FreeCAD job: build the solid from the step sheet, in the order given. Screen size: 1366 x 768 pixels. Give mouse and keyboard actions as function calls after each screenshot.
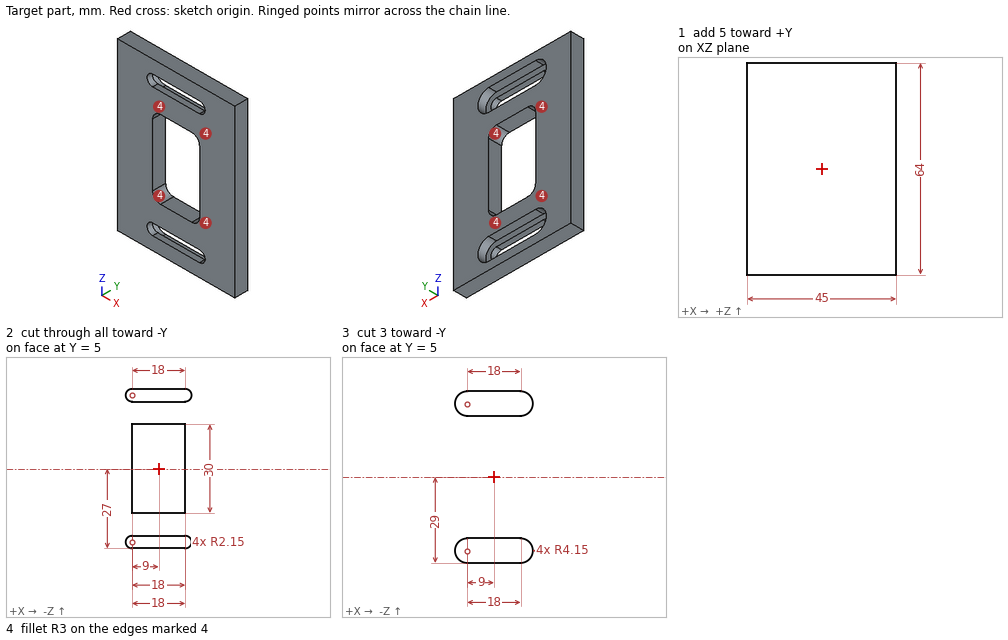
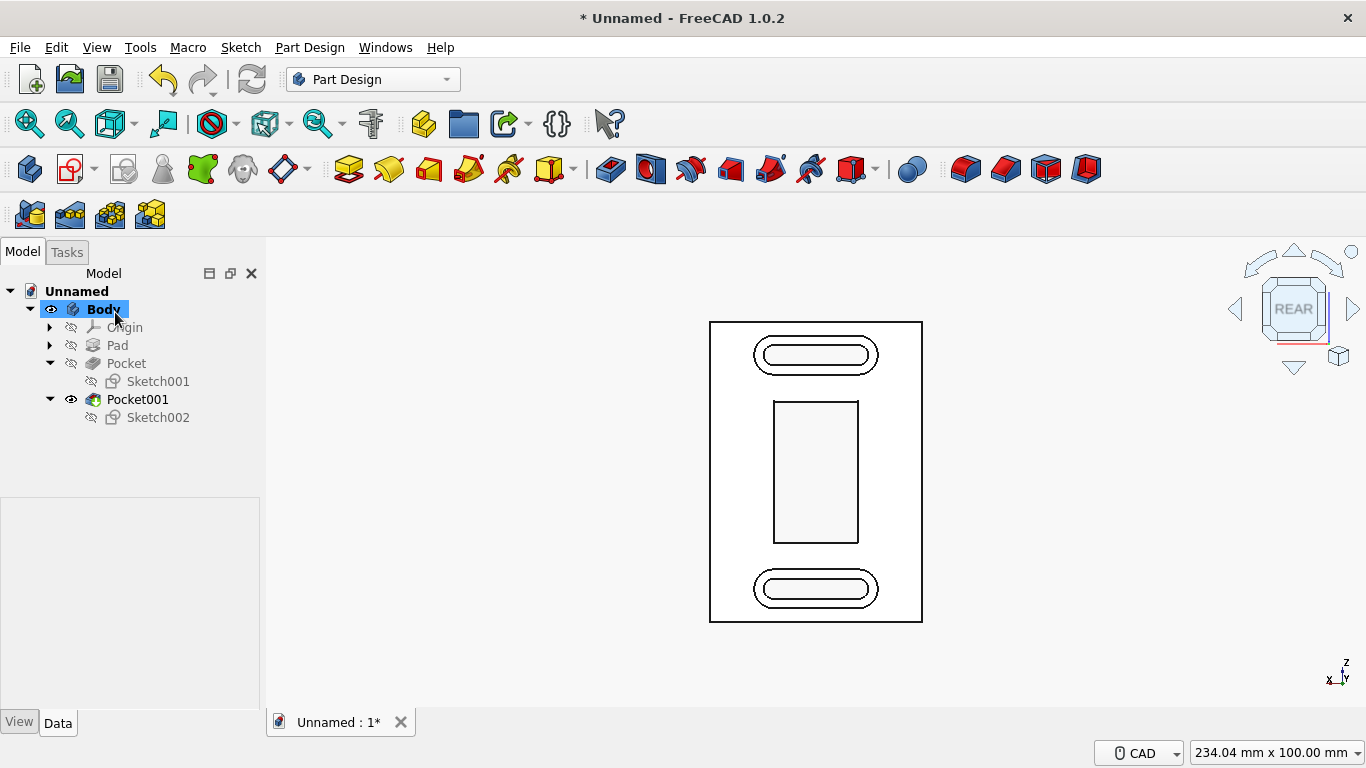
key(0)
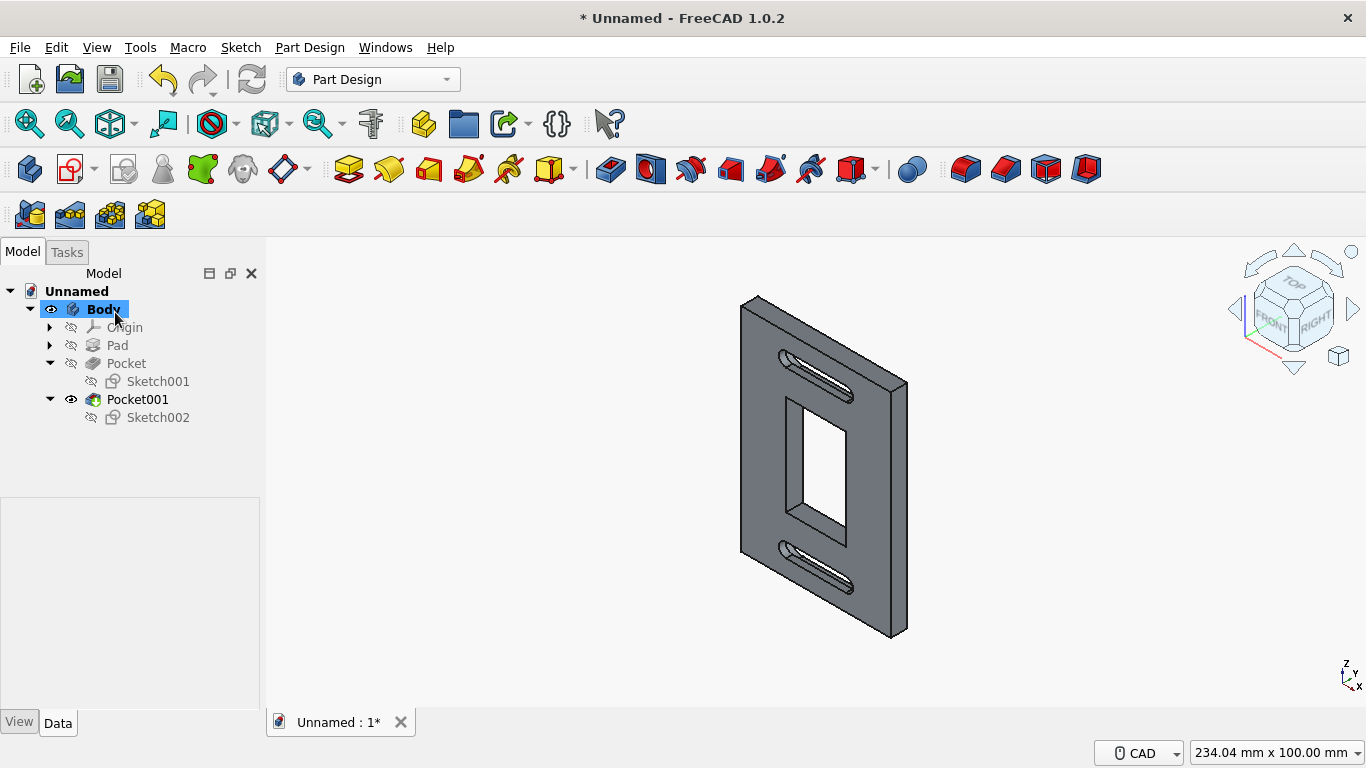
key(2)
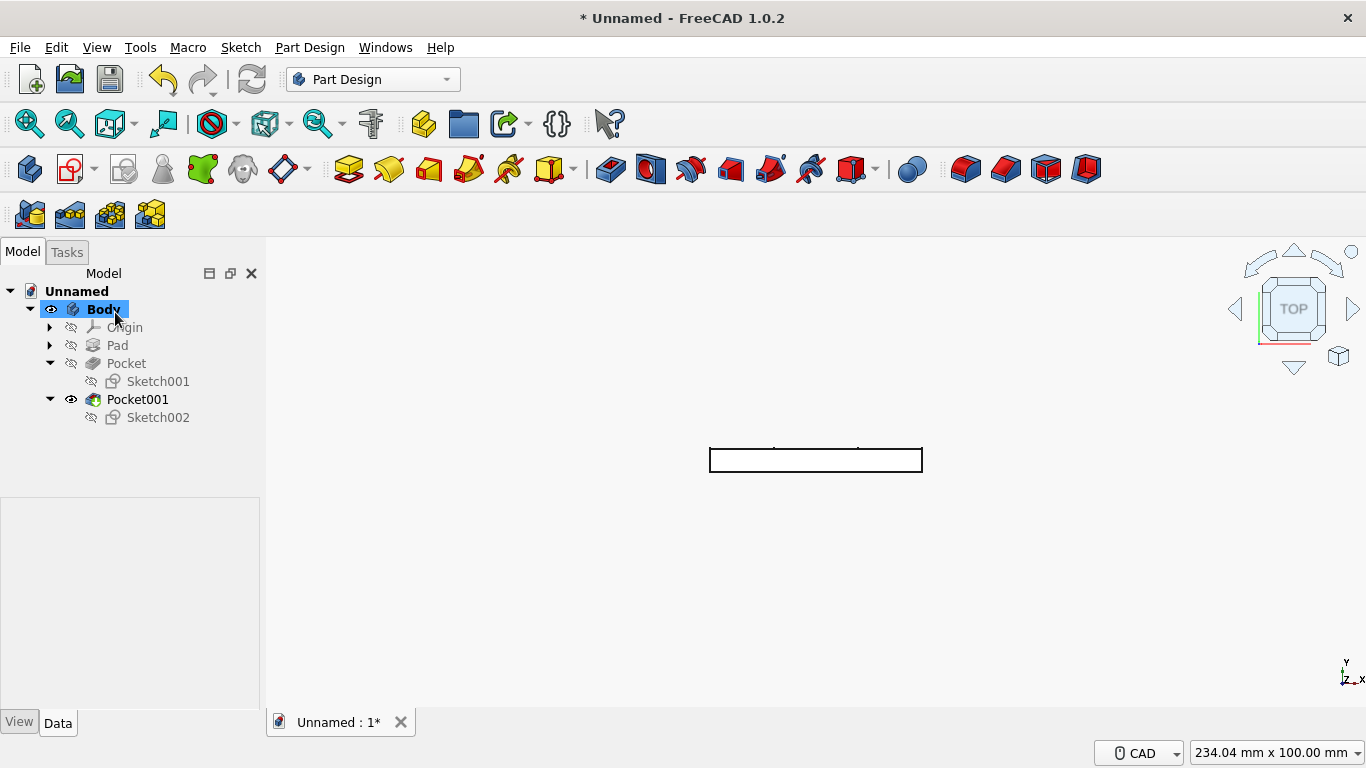
click(30, 124)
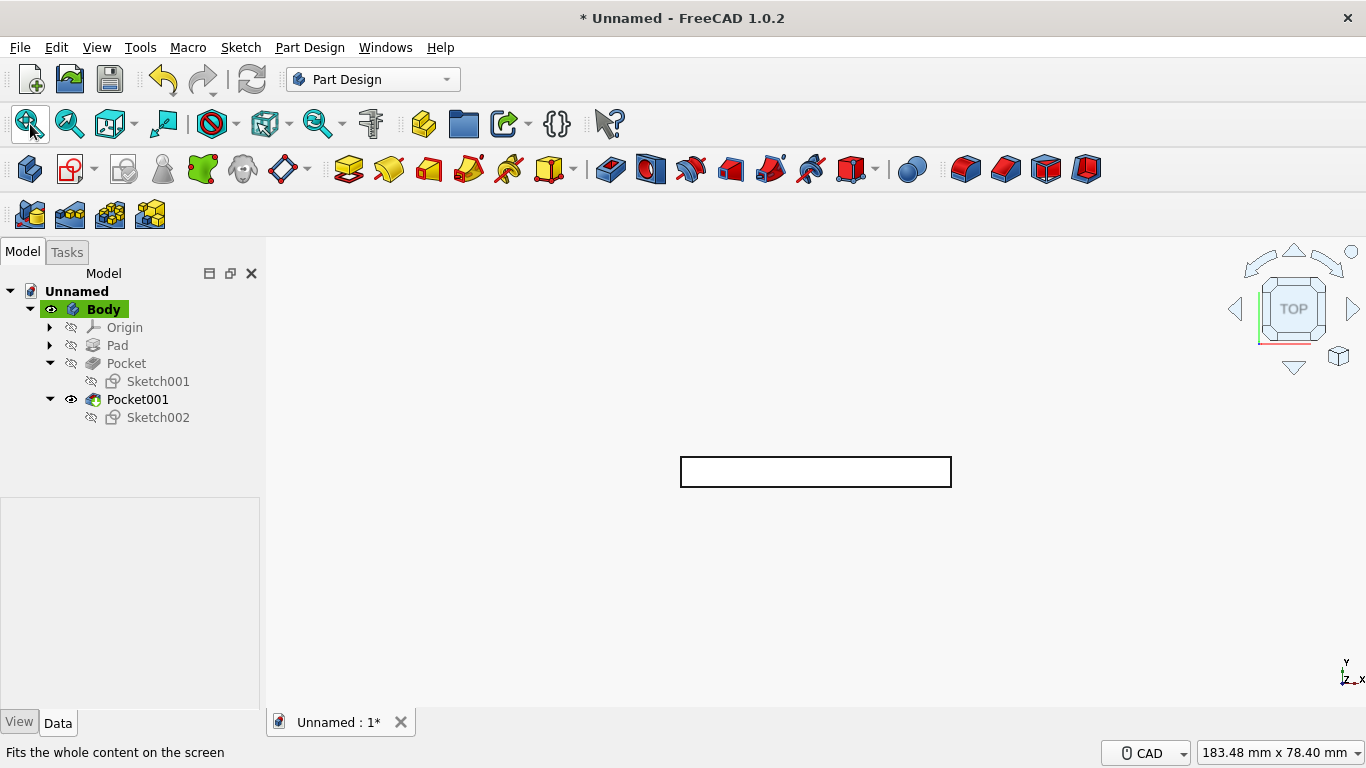
key(1)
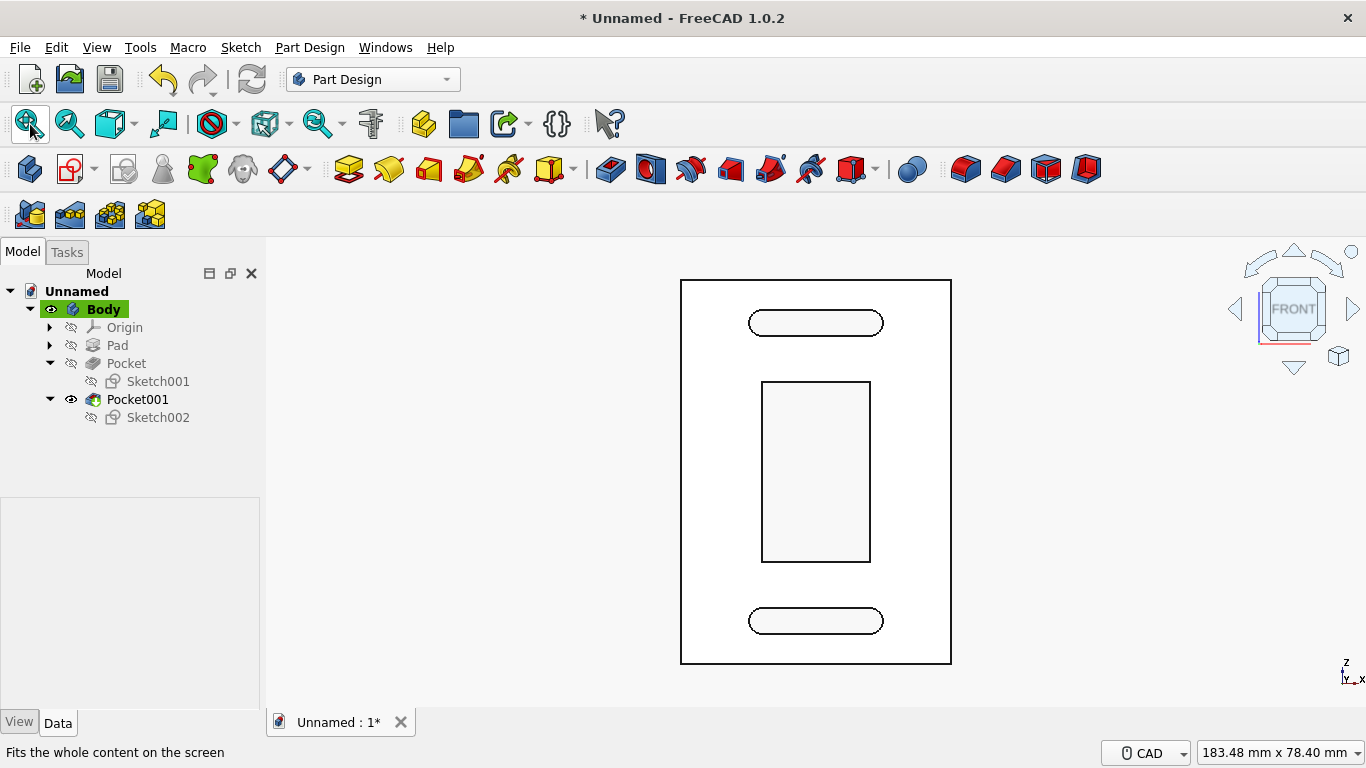
key(3)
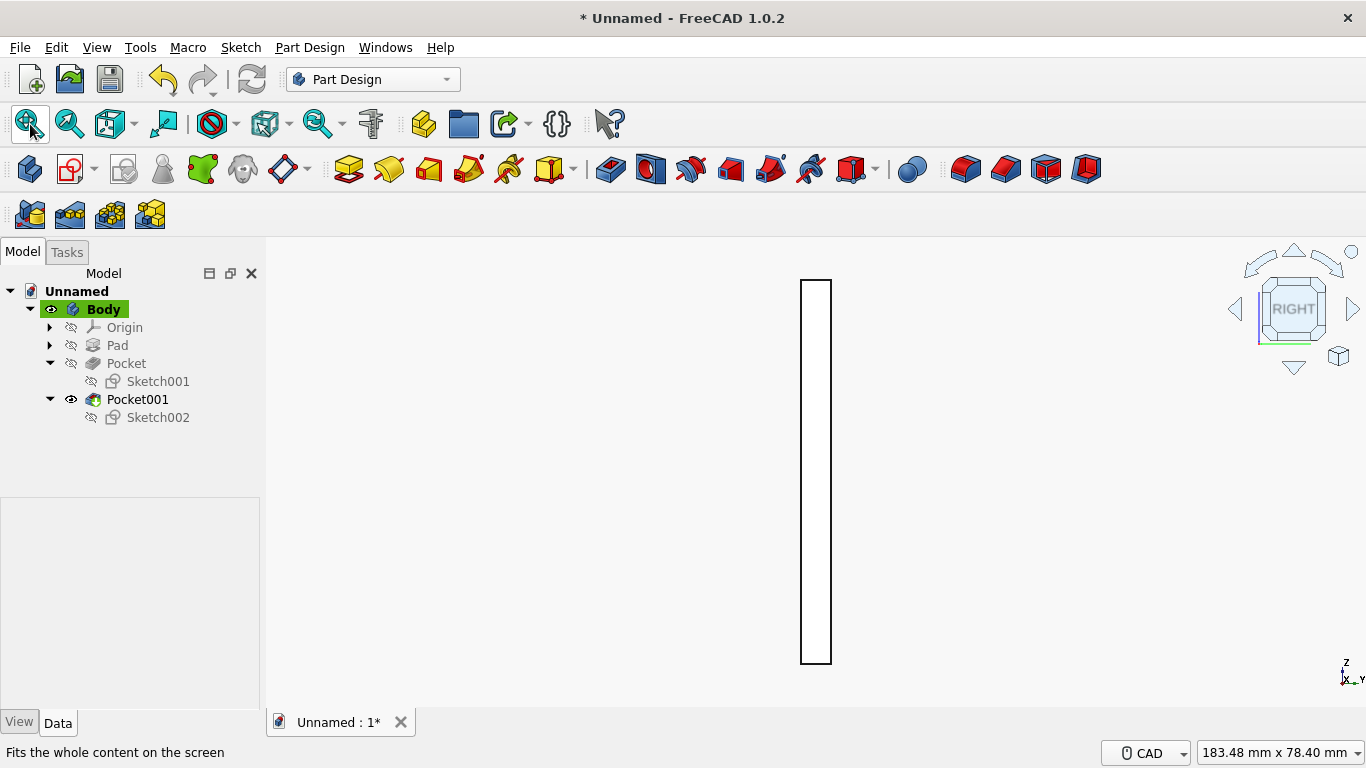
key(5)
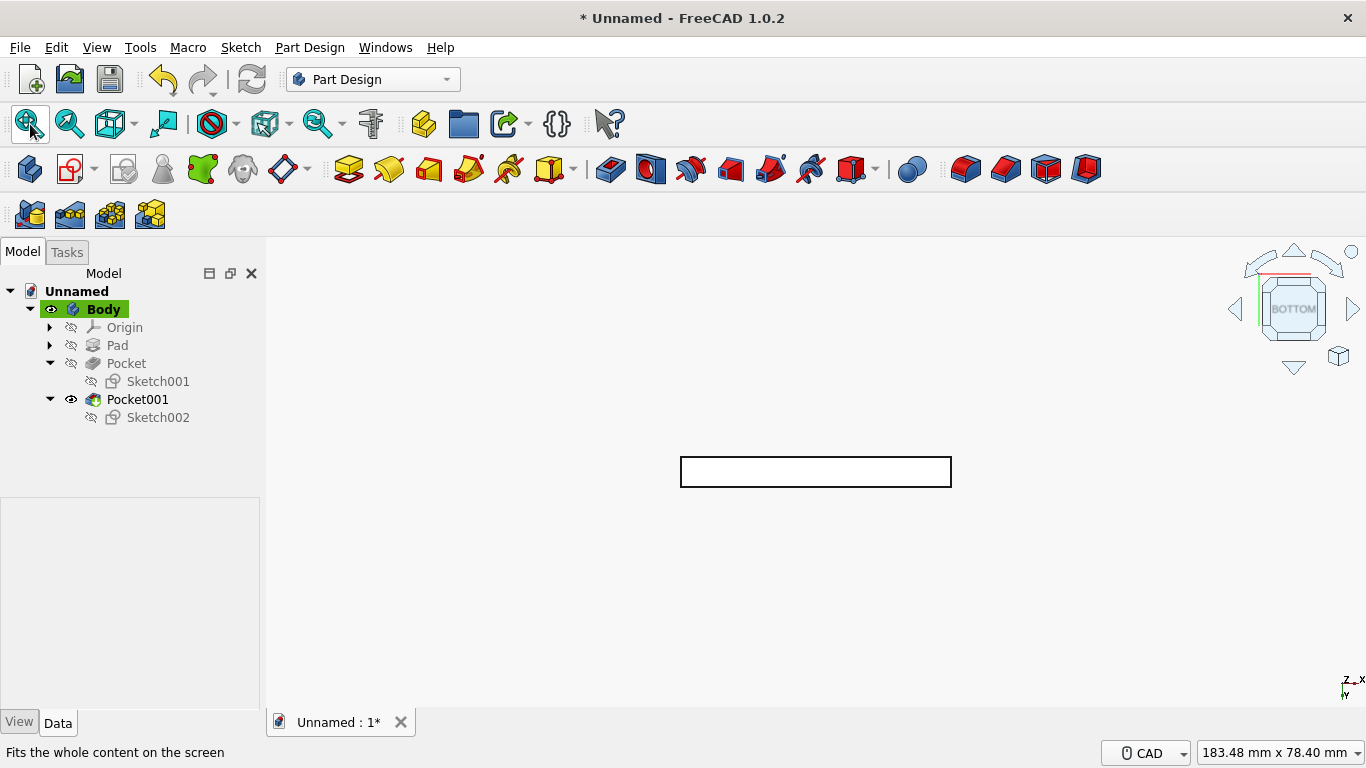
click(30, 124)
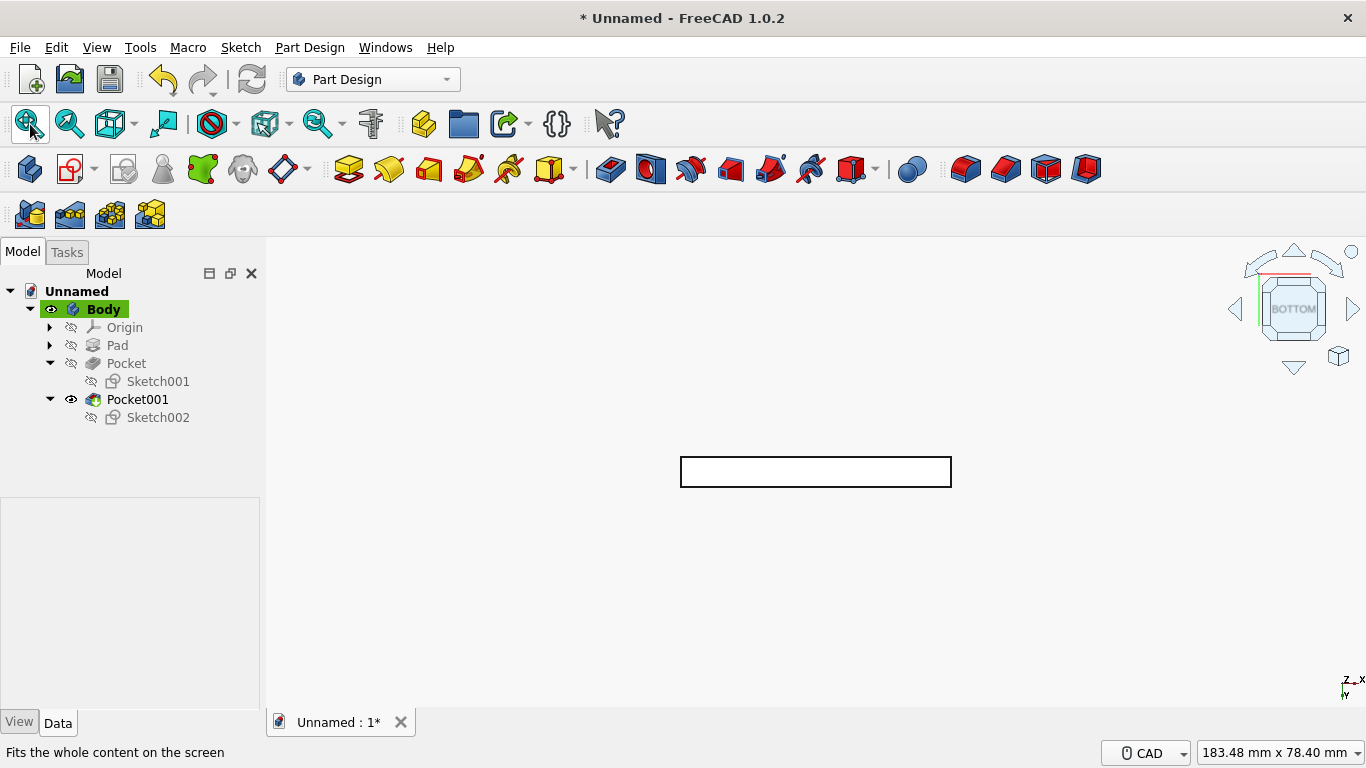
key(4)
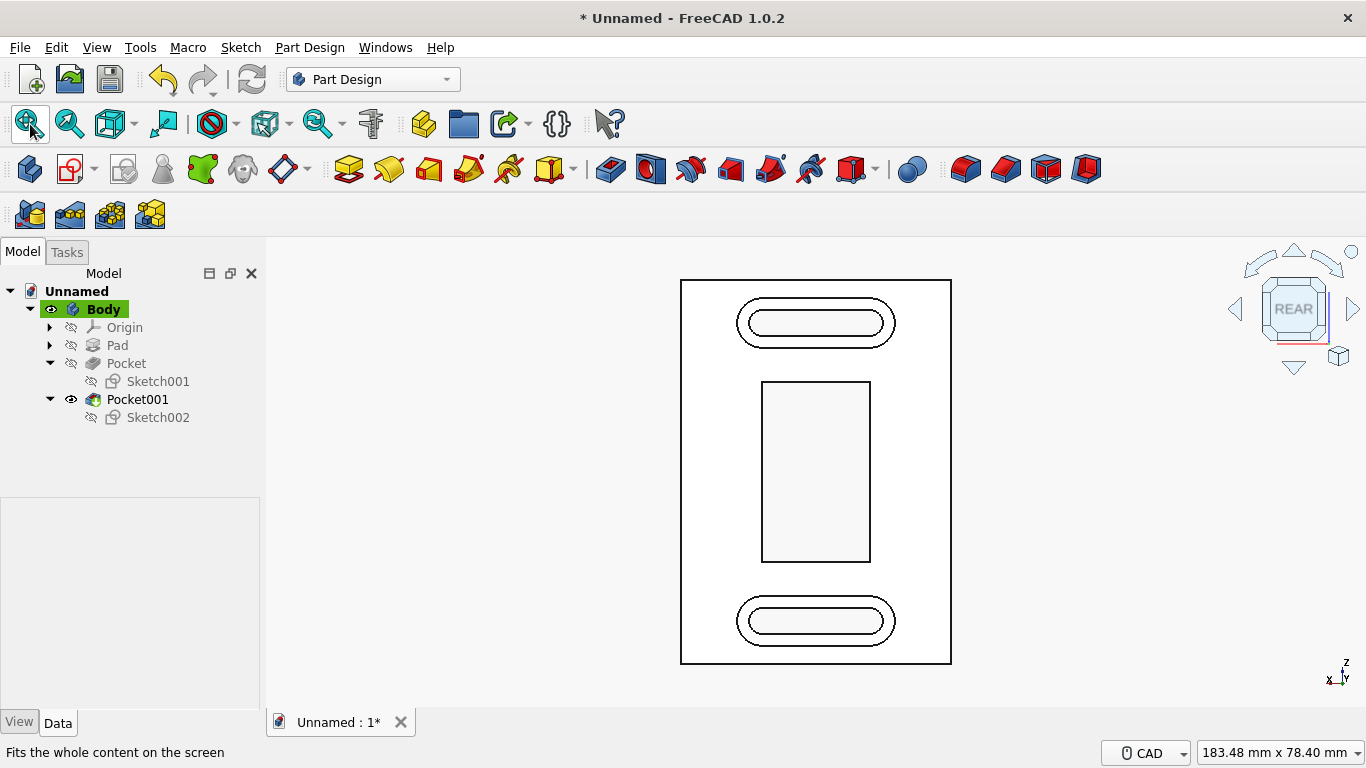
key(6)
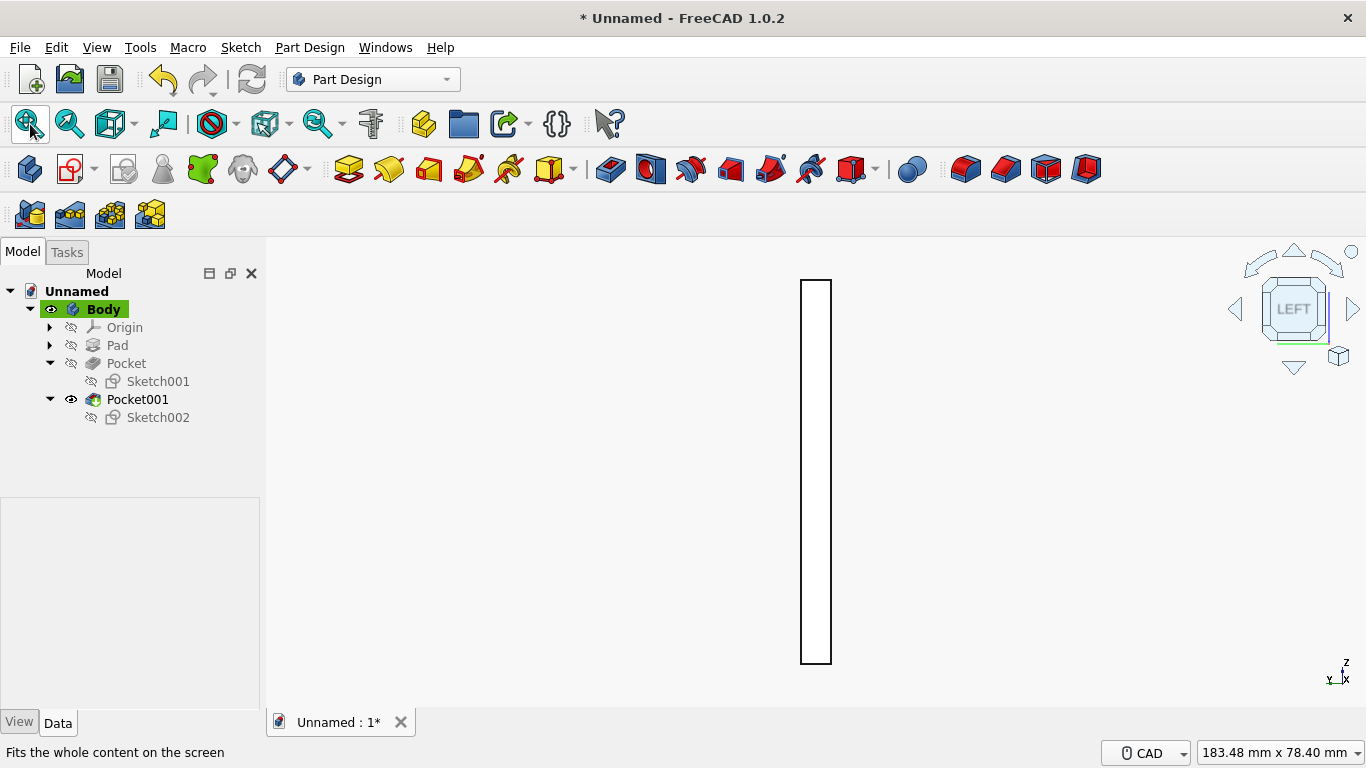
key(v)
key(3)